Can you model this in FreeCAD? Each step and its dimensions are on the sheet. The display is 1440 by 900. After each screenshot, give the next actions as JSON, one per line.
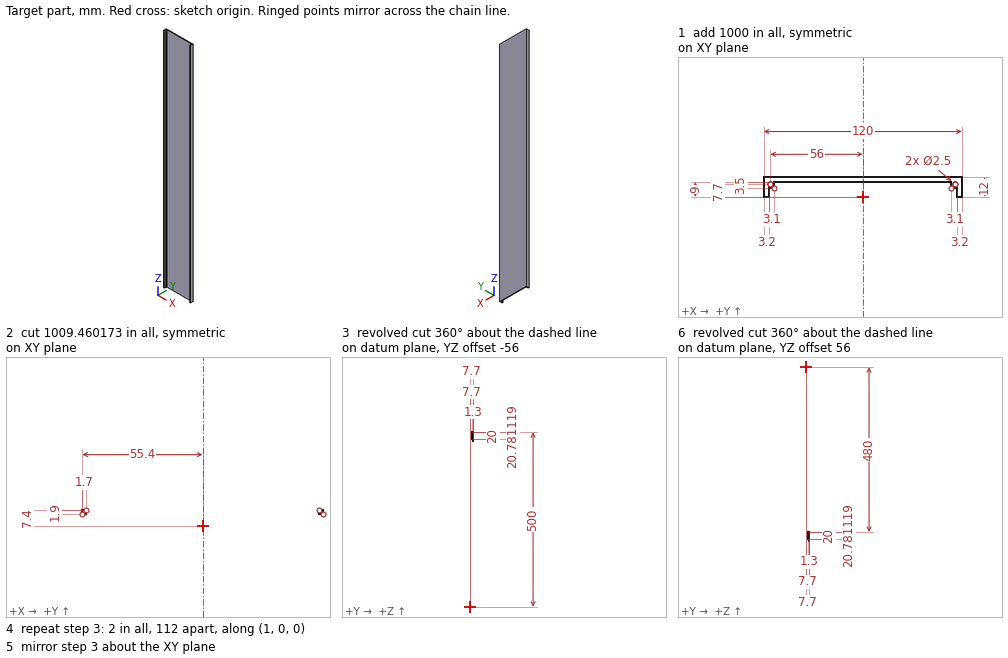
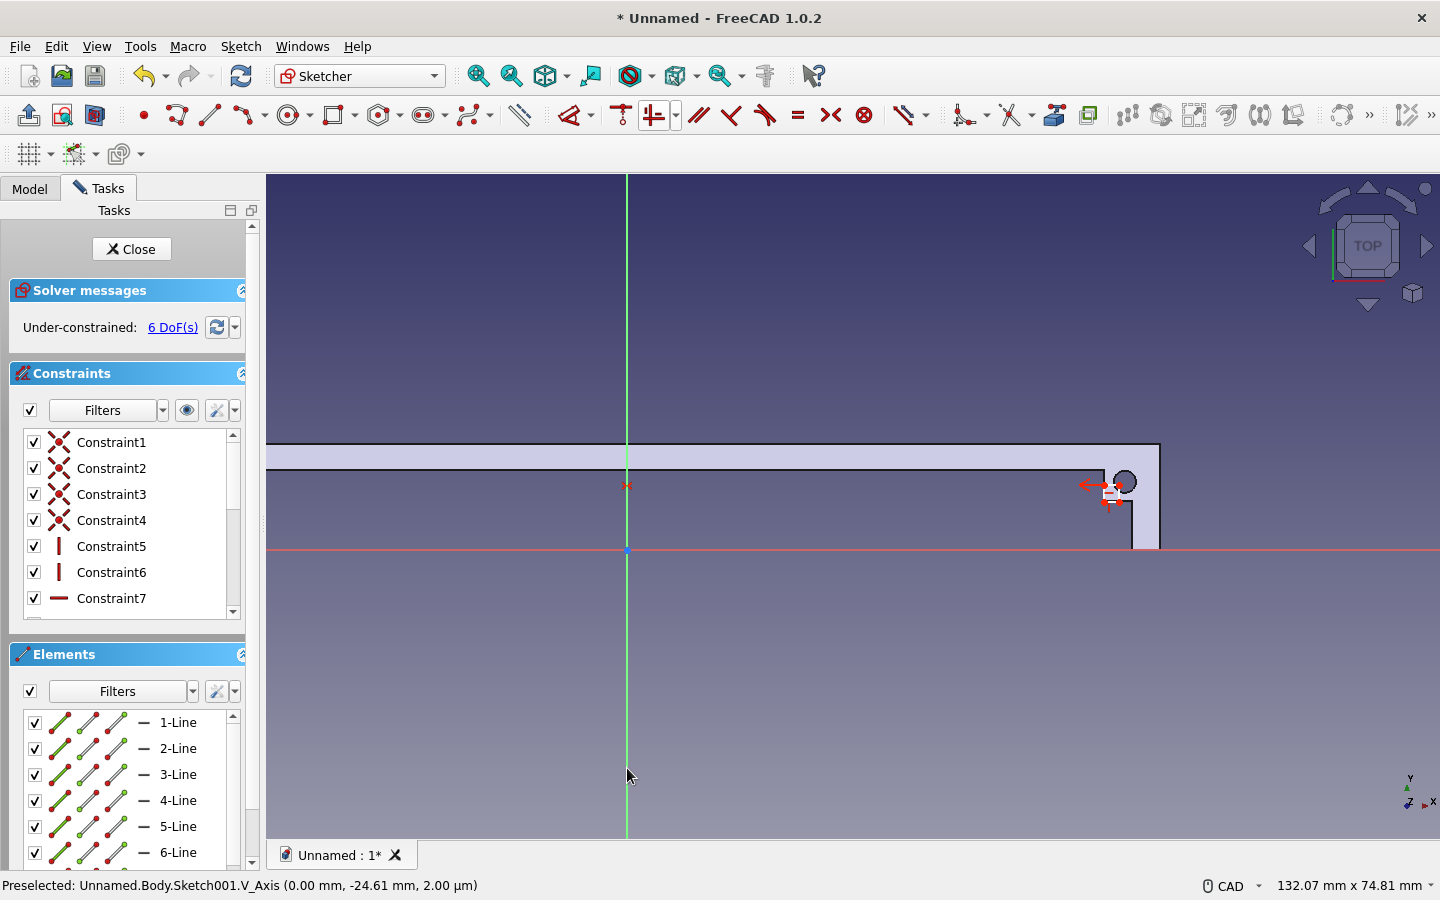
{"action": "scroll", "coordinate": [1105, 484], "scroll_direction": "down", "scroll_amount": 2}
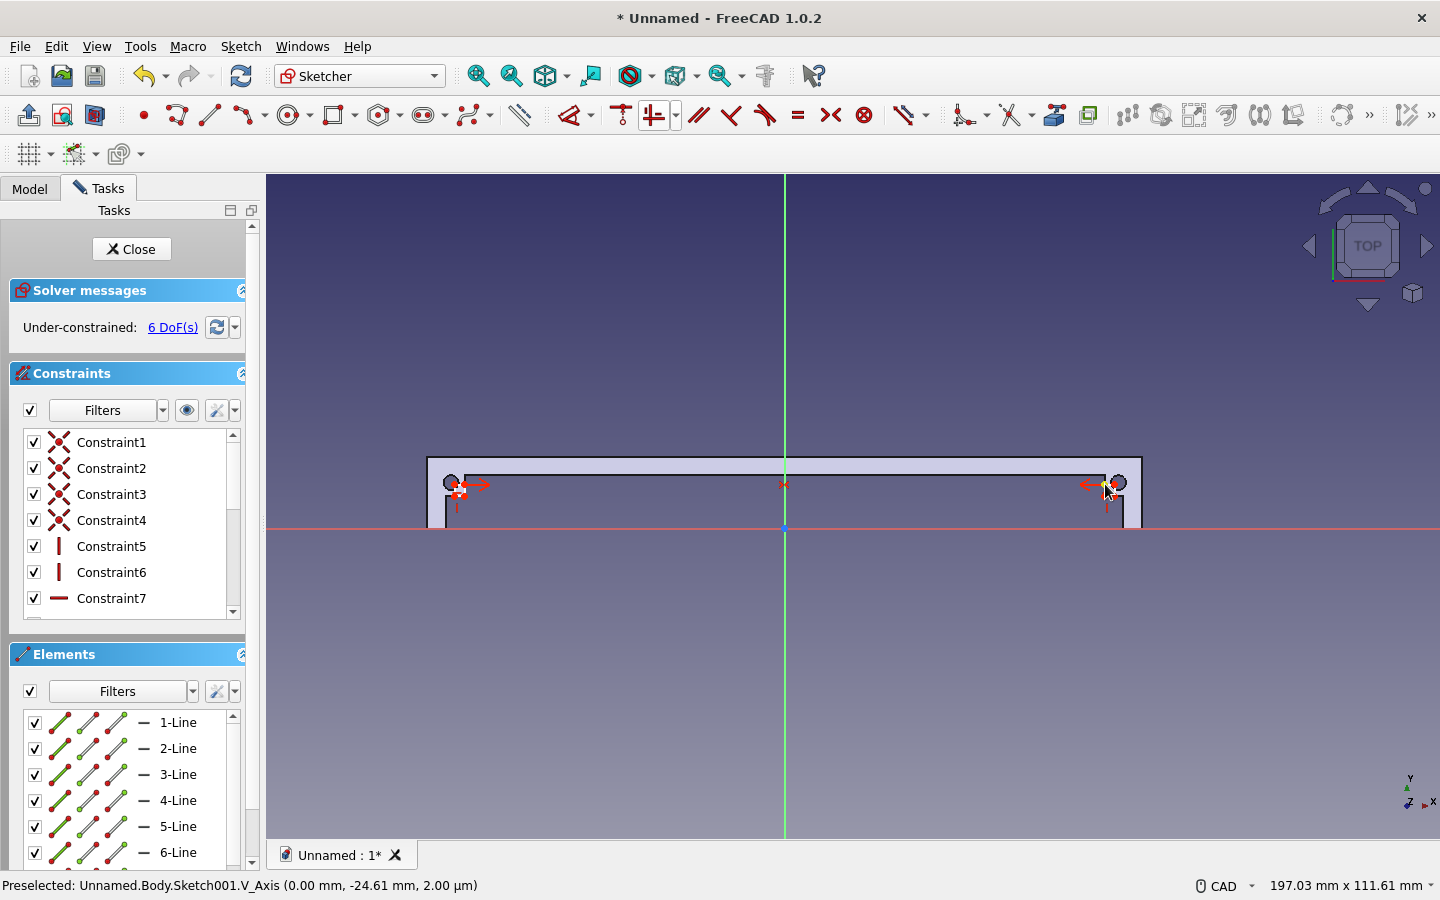
{"action": "left_click", "coordinate": [455, 496]}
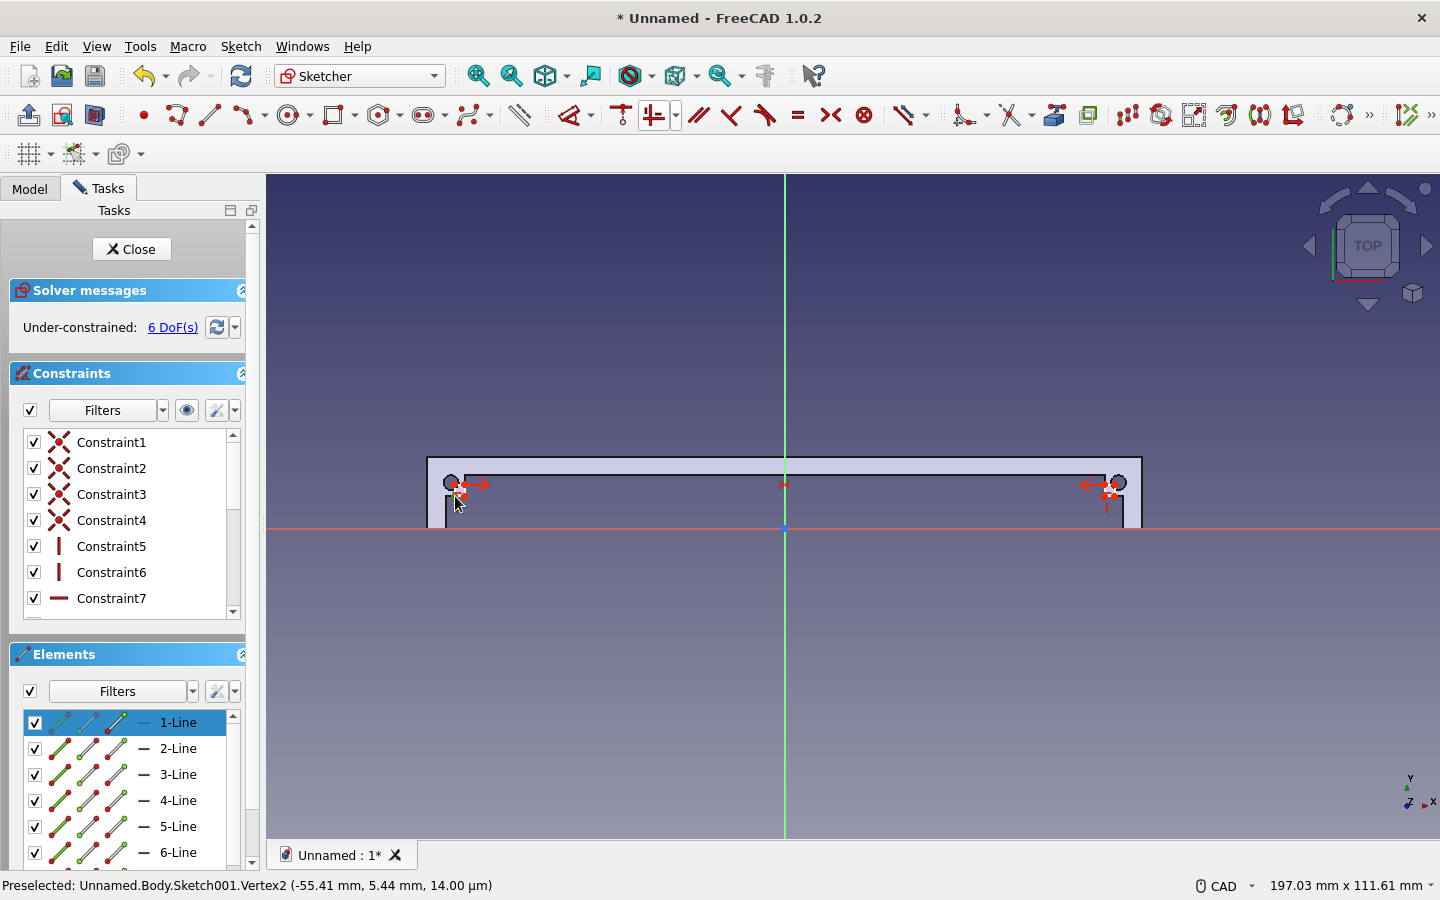
{"action": "scroll", "coordinate": [1115, 496], "scroll_direction": "up", "scroll_amount": 2}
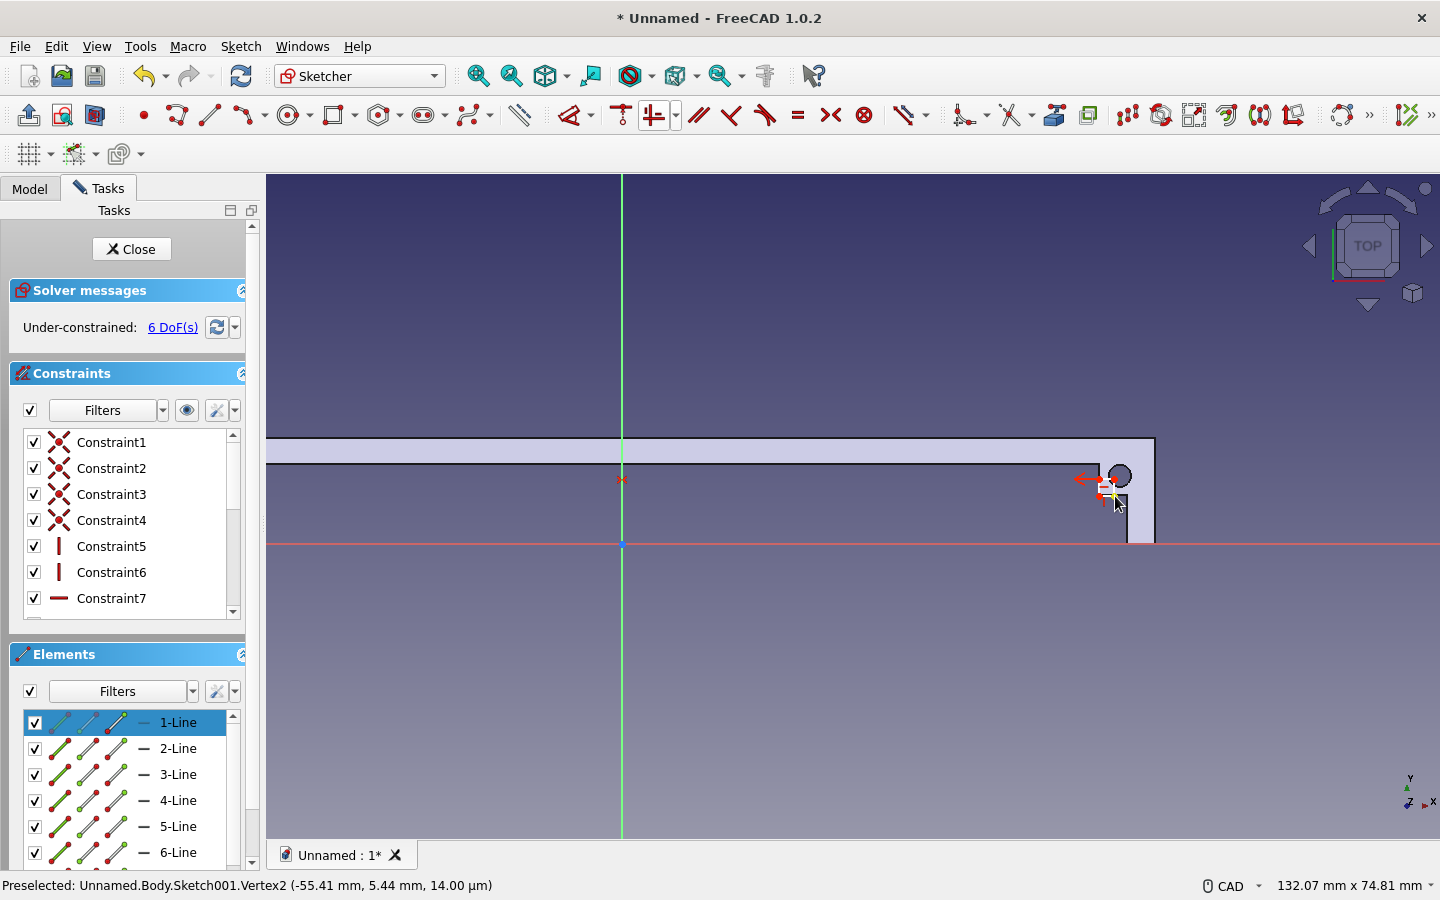
{"action": "left_click", "coordinate": [1114, 496]}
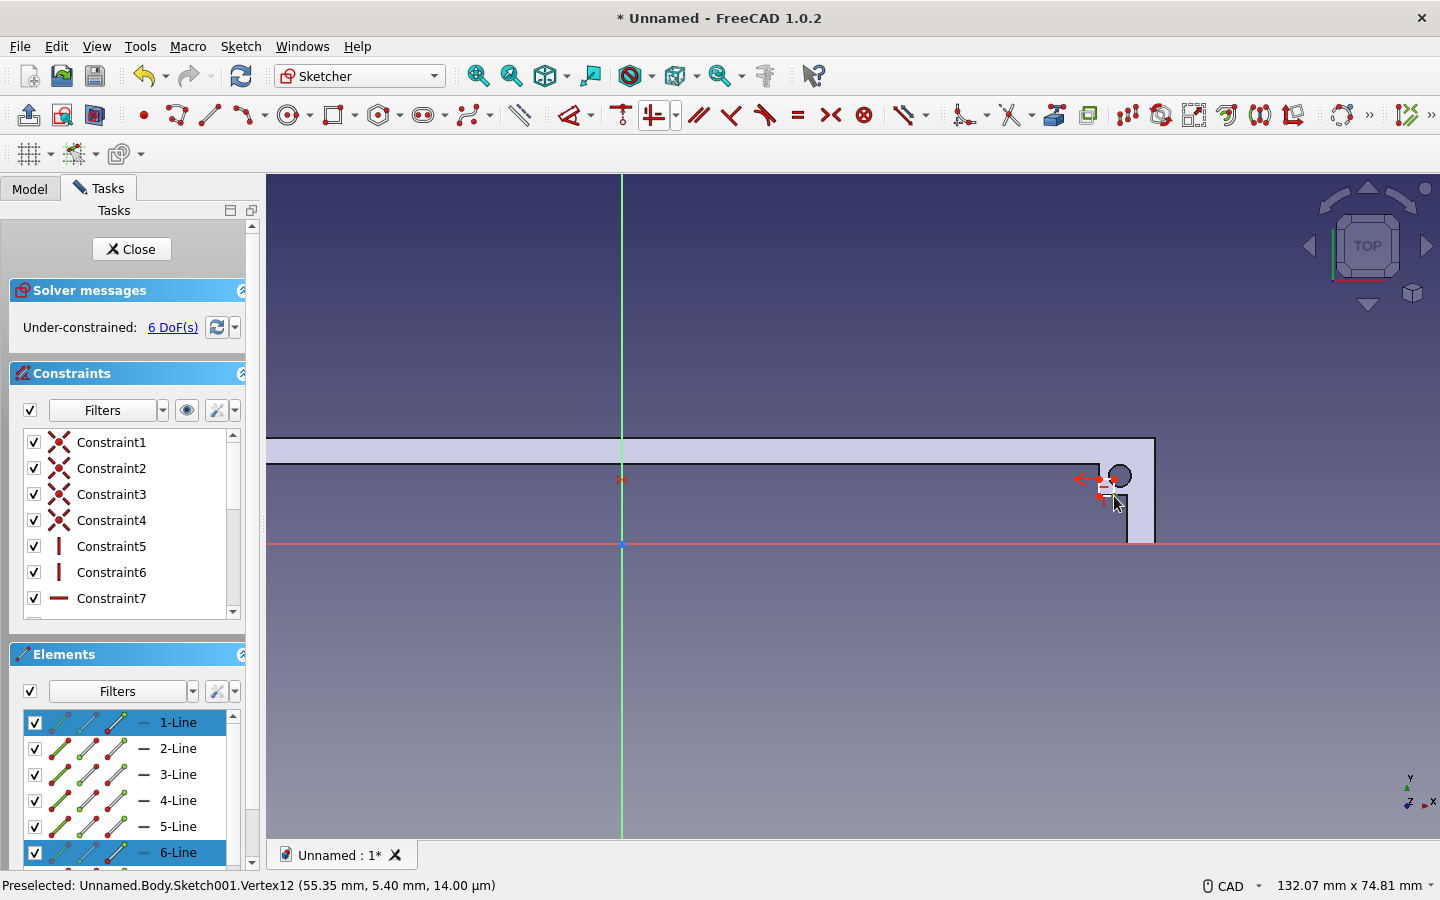
{"action": "left_click", "coordinate": [622, 768]}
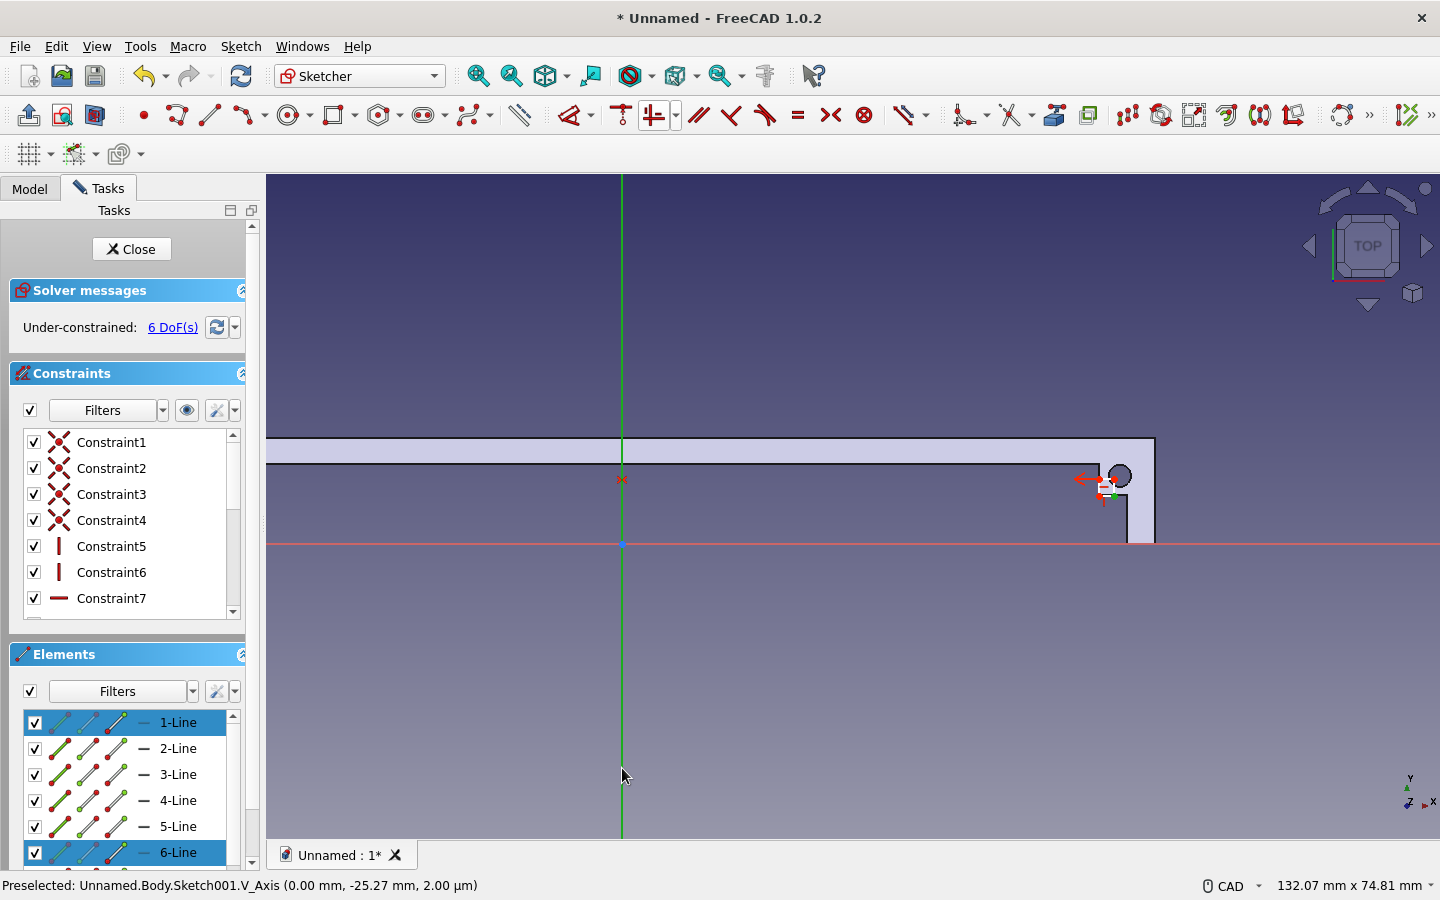
{"action": "key", "text": "s"}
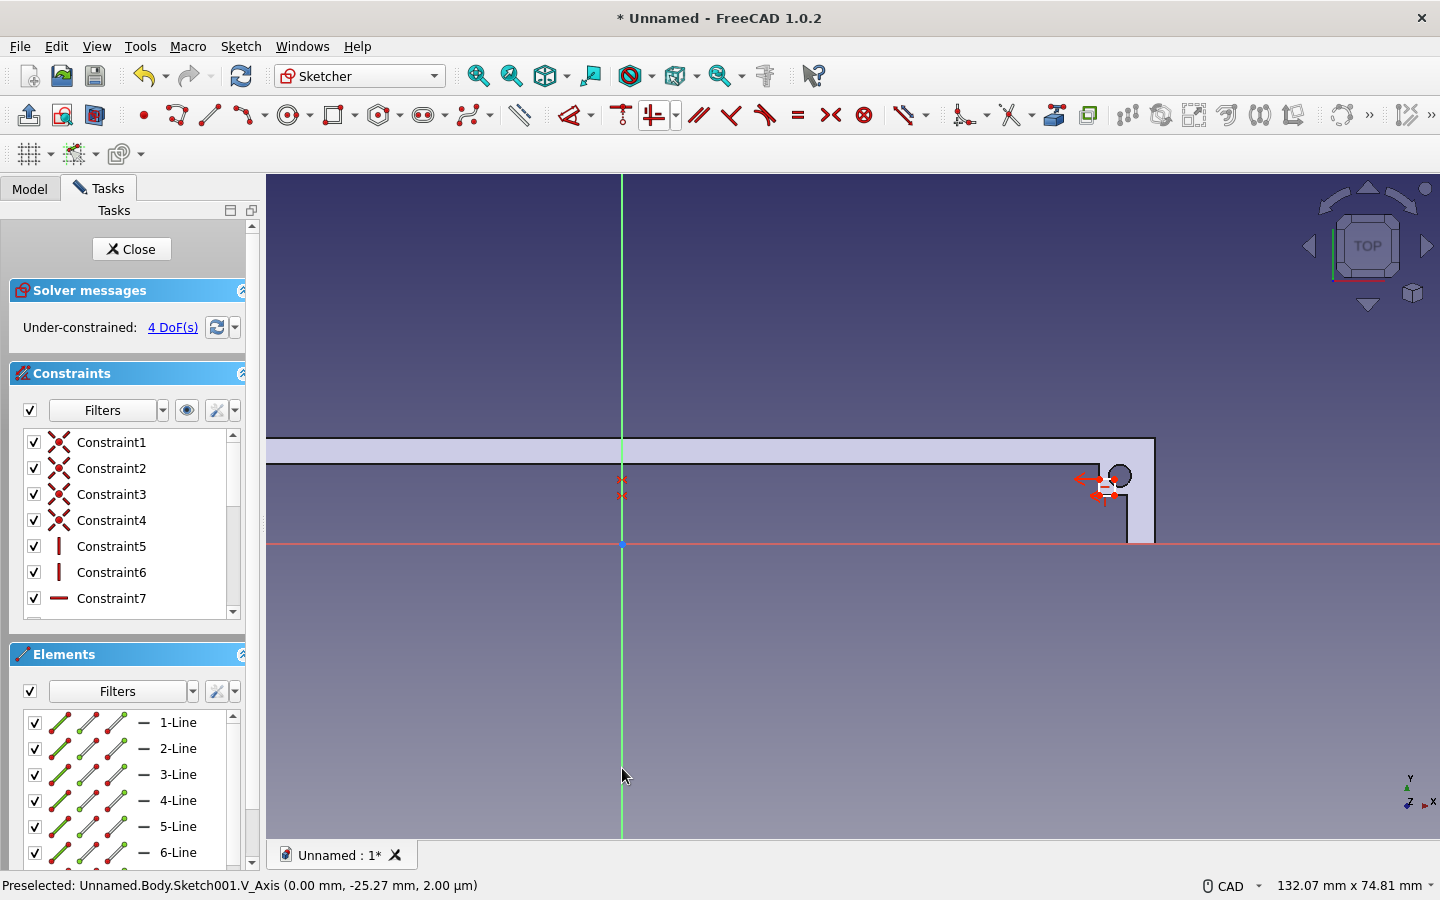
{"action": "key", "text": "d"}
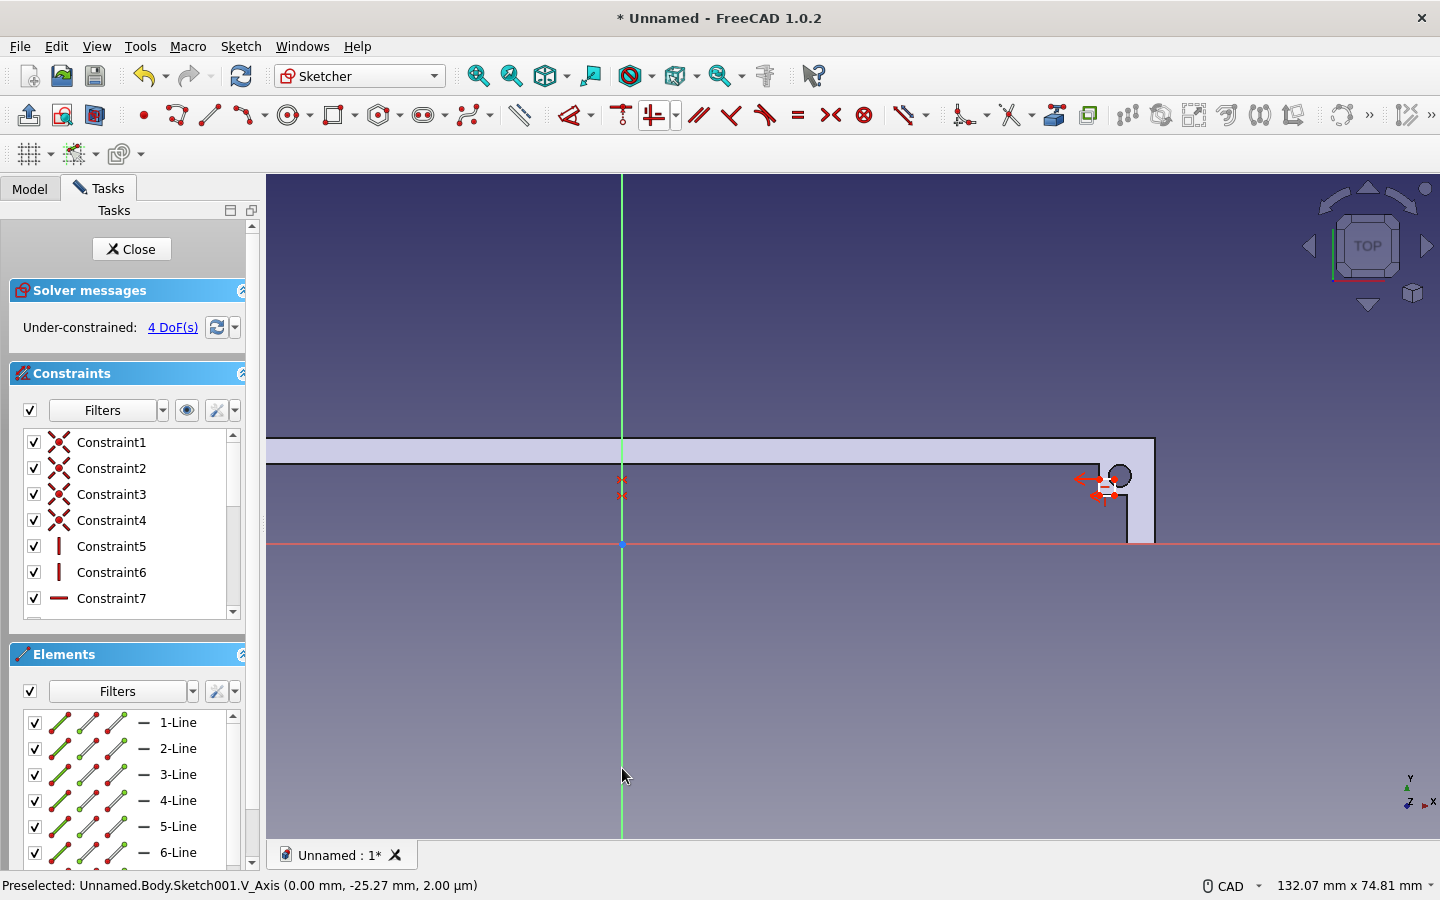
{"action": "scroll", "coordinate": [1115, 496], "scroll_direction": "down", "scroll_amount": 2}